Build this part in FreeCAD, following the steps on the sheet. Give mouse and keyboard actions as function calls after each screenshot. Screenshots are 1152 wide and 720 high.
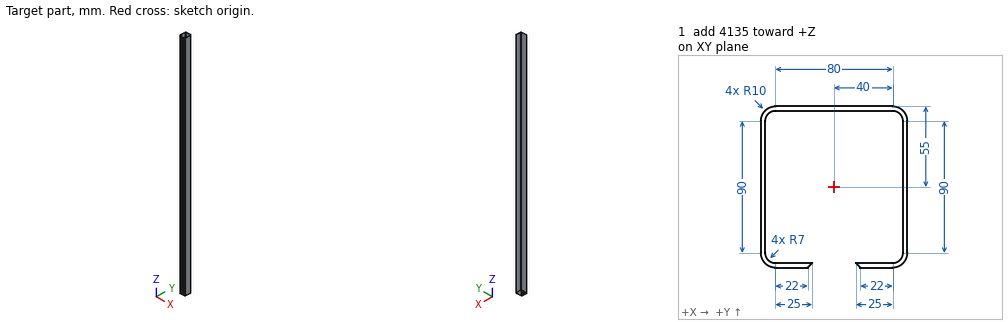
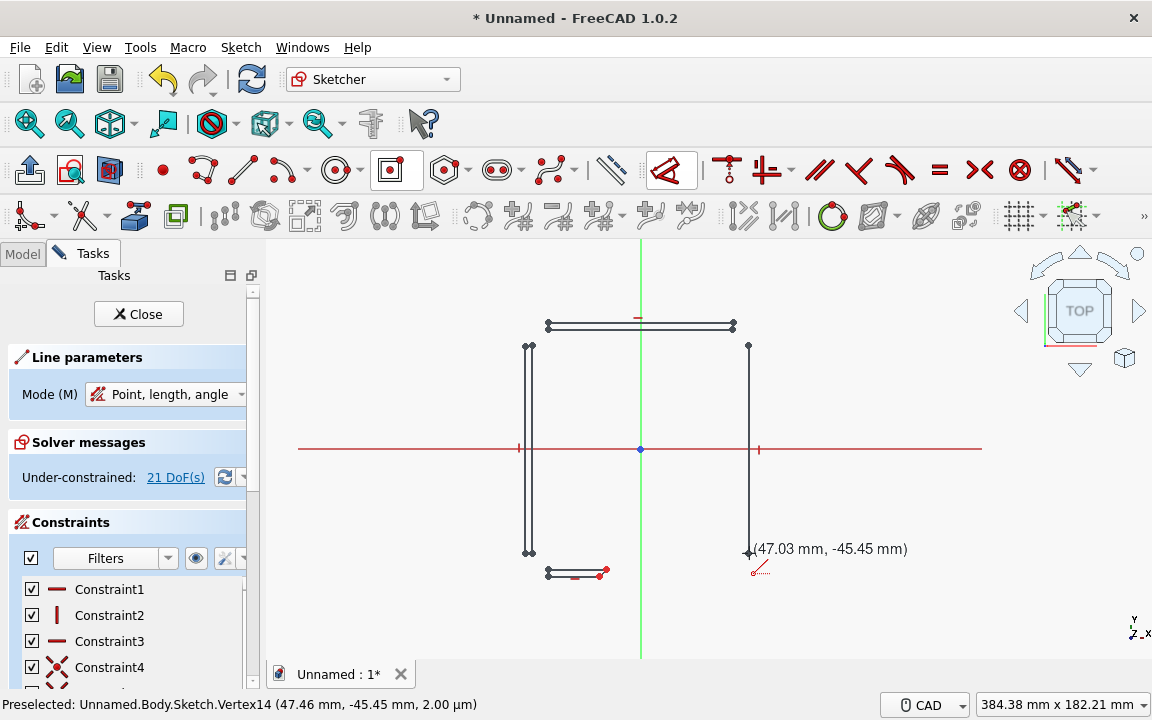
click(204, 170)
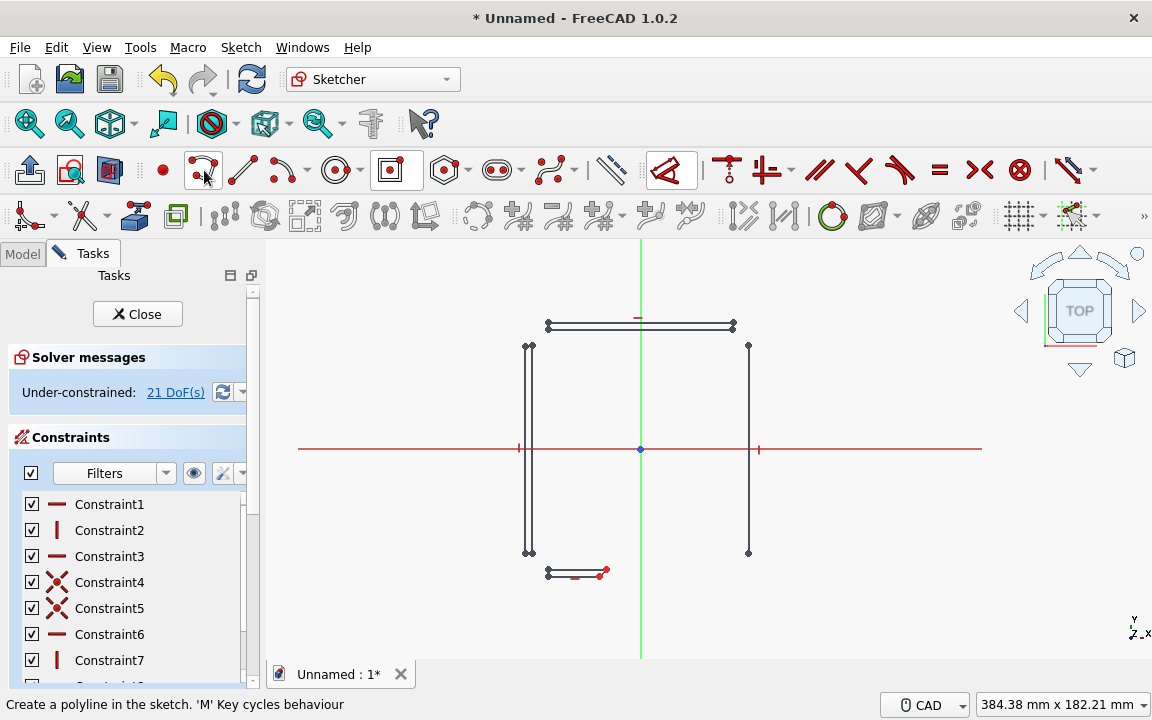
click(733, 569)
click(675, 569)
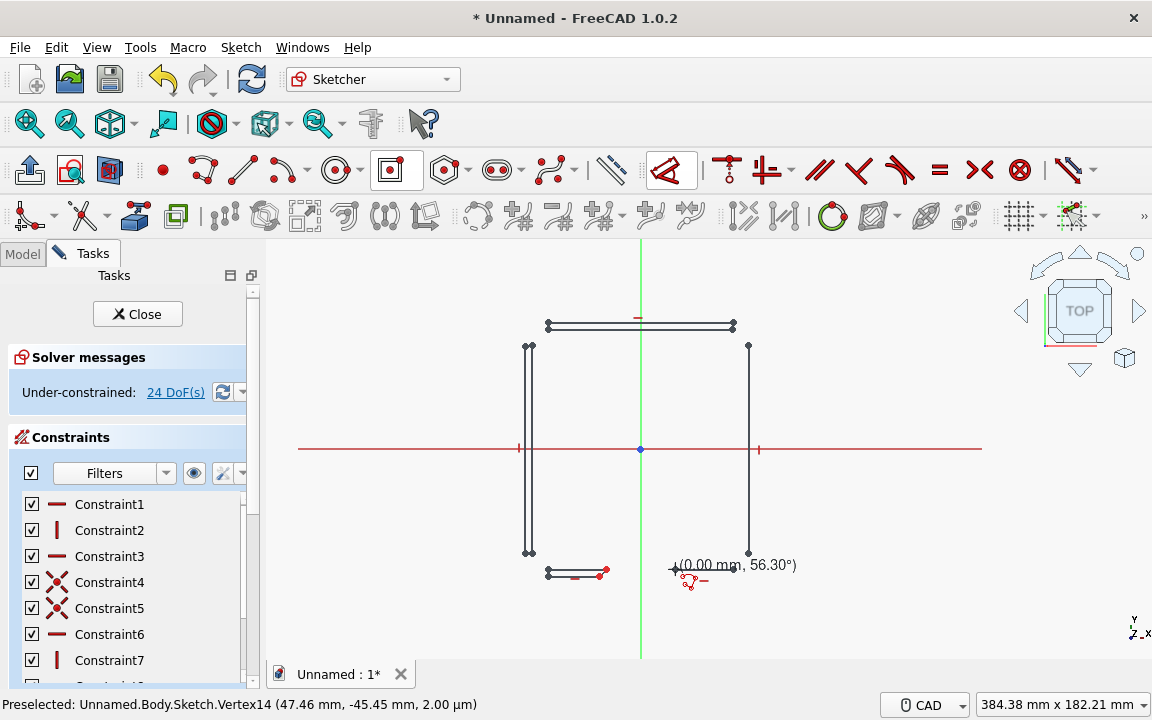
scroll(682, 576, up, 5)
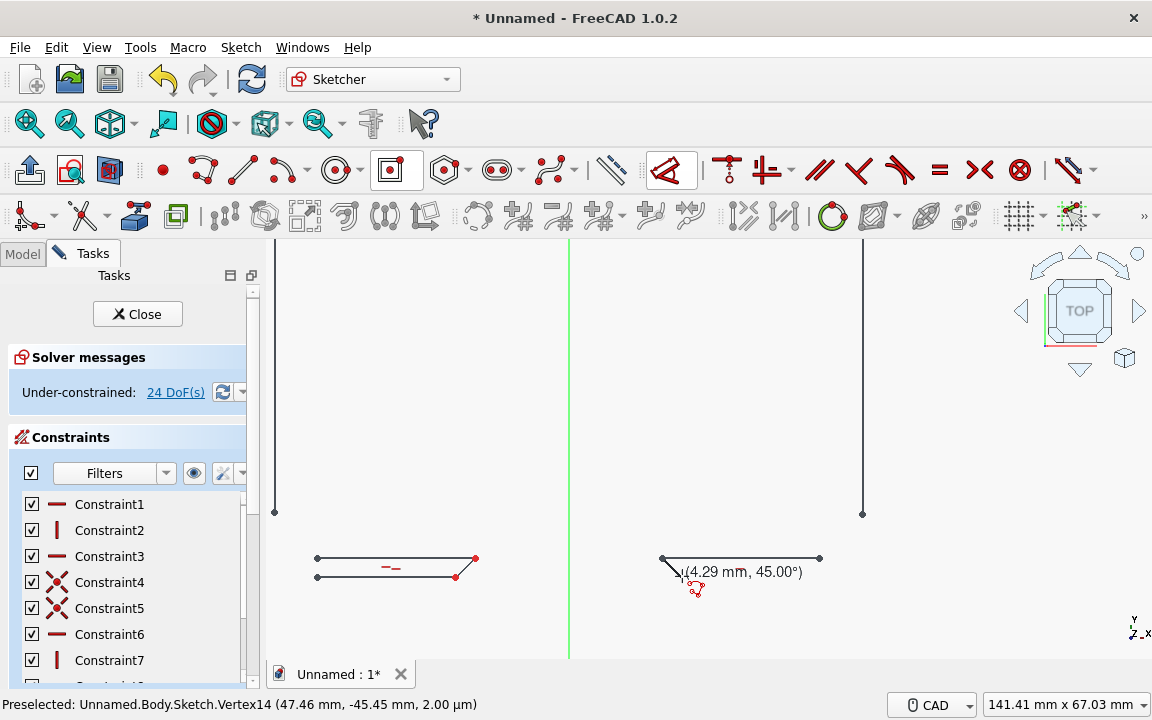
click(681, 575)
click(819, 575)
right_click(819, 575)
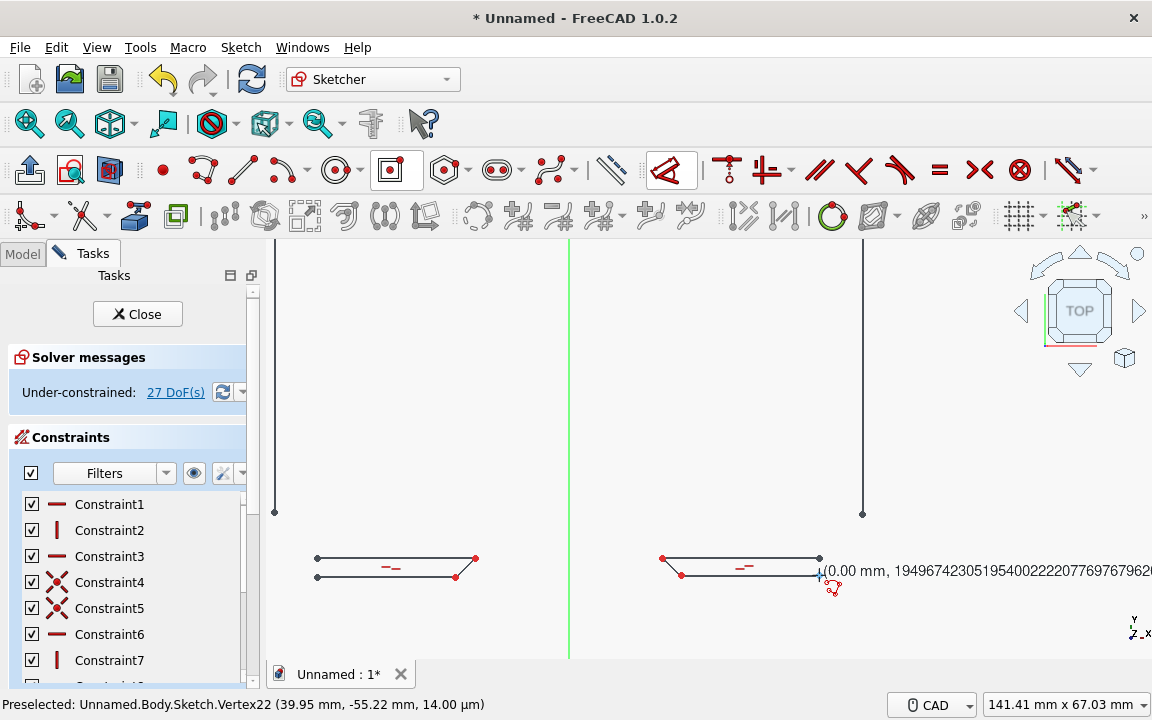
click(244, 170)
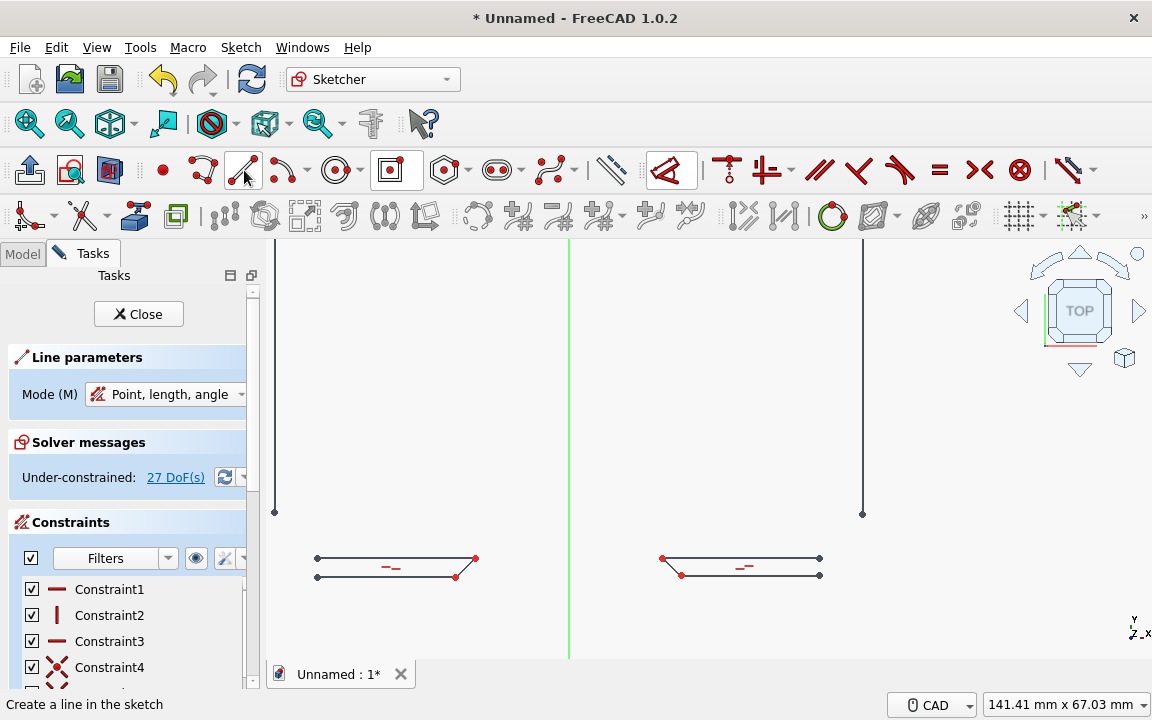
click(882, 512)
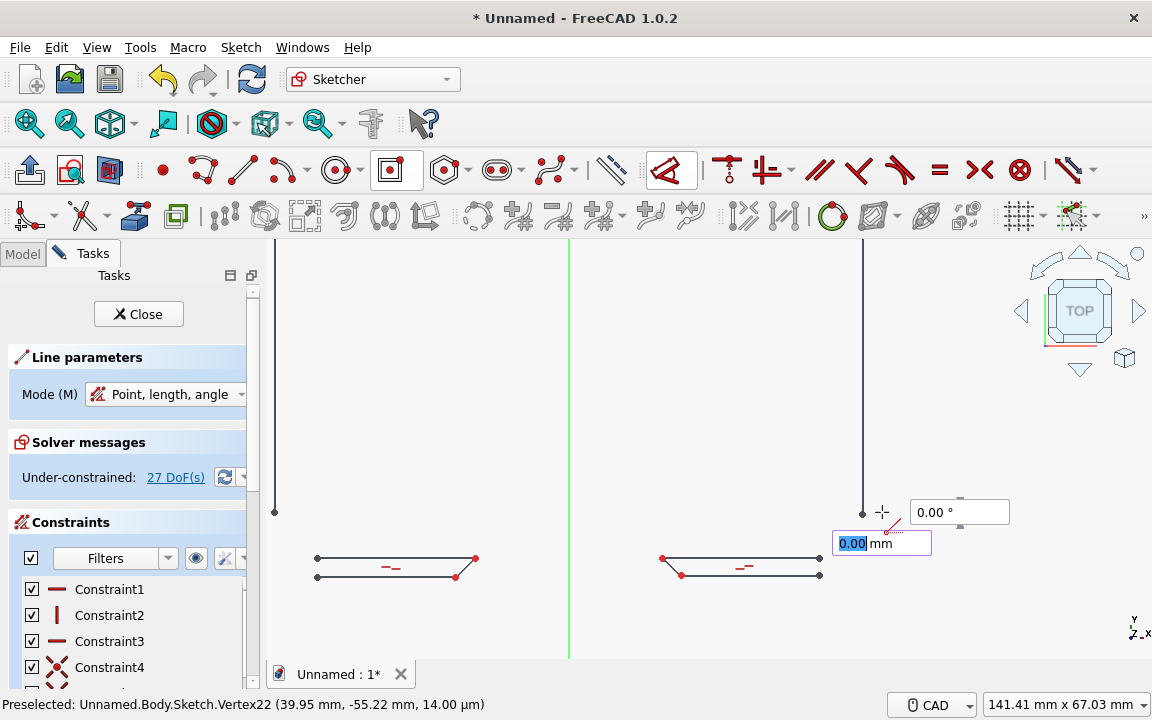
scroll(682, 576, down, 5)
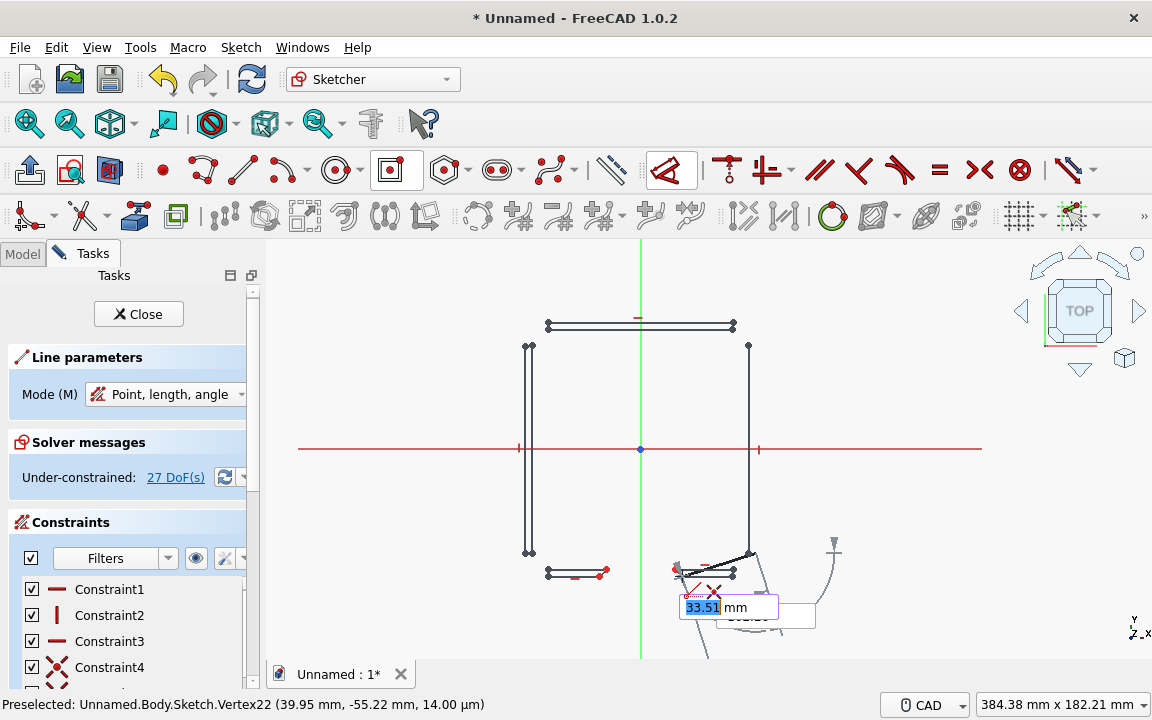
scroll(756, 346, up, 5)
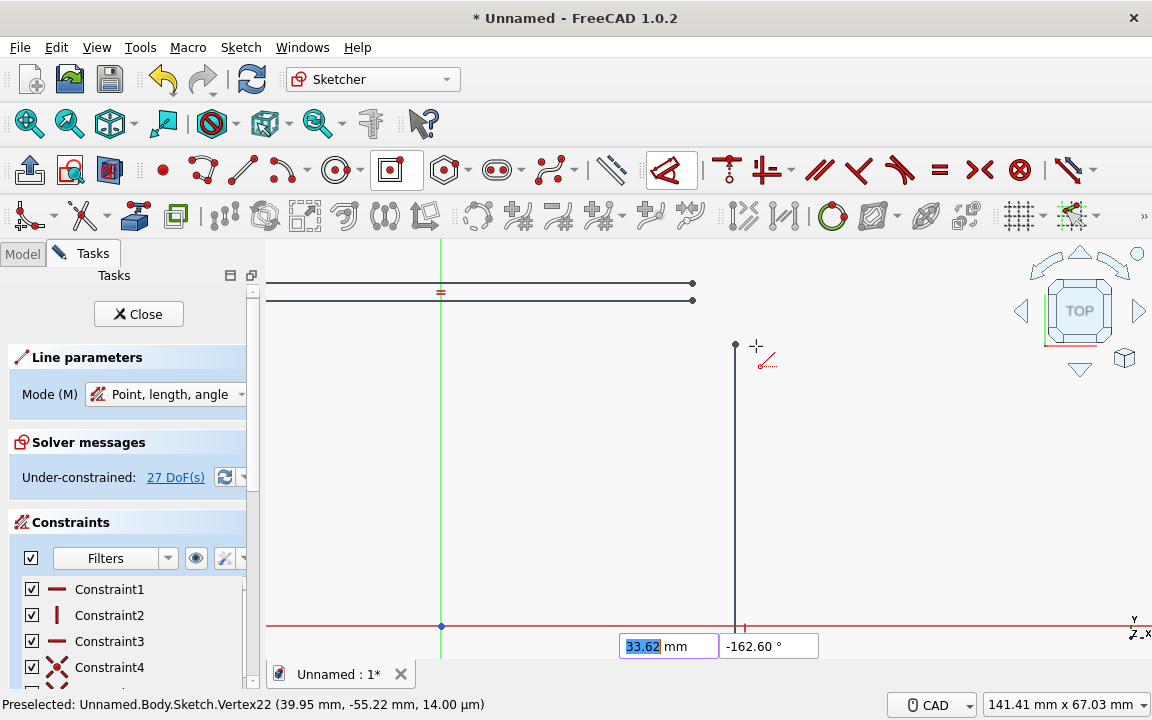
click(755, 344)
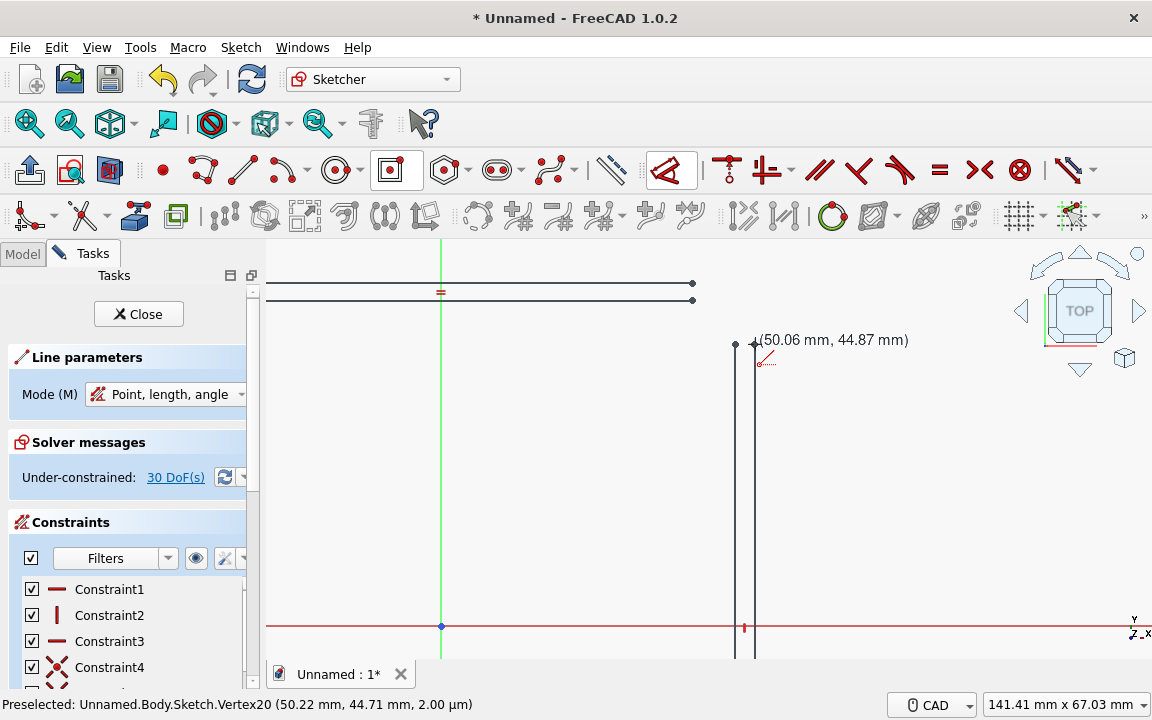
click(310, 170)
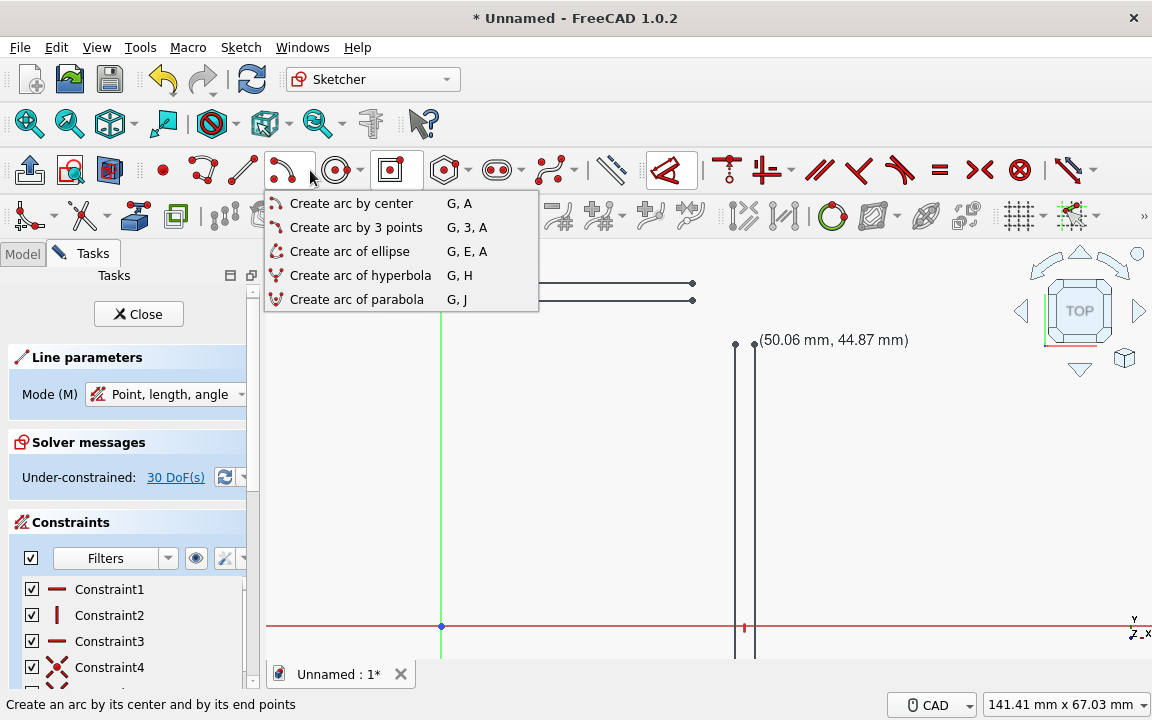
click(402, 227)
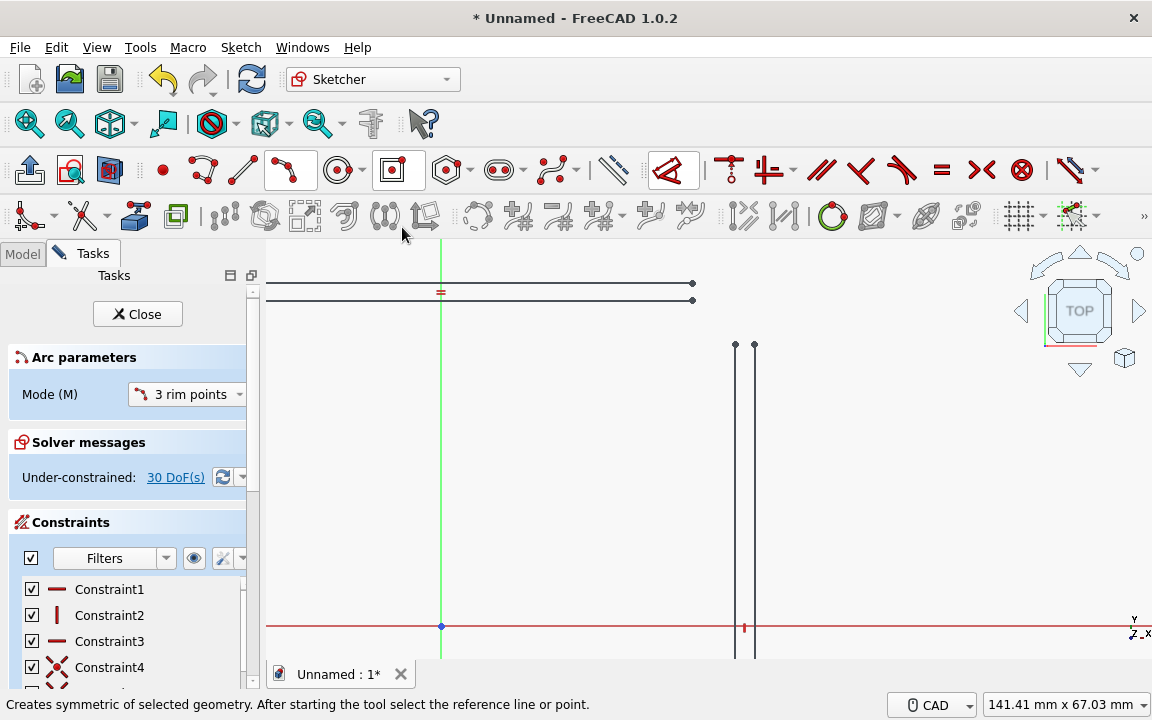
scroll(756, 346, down, 5)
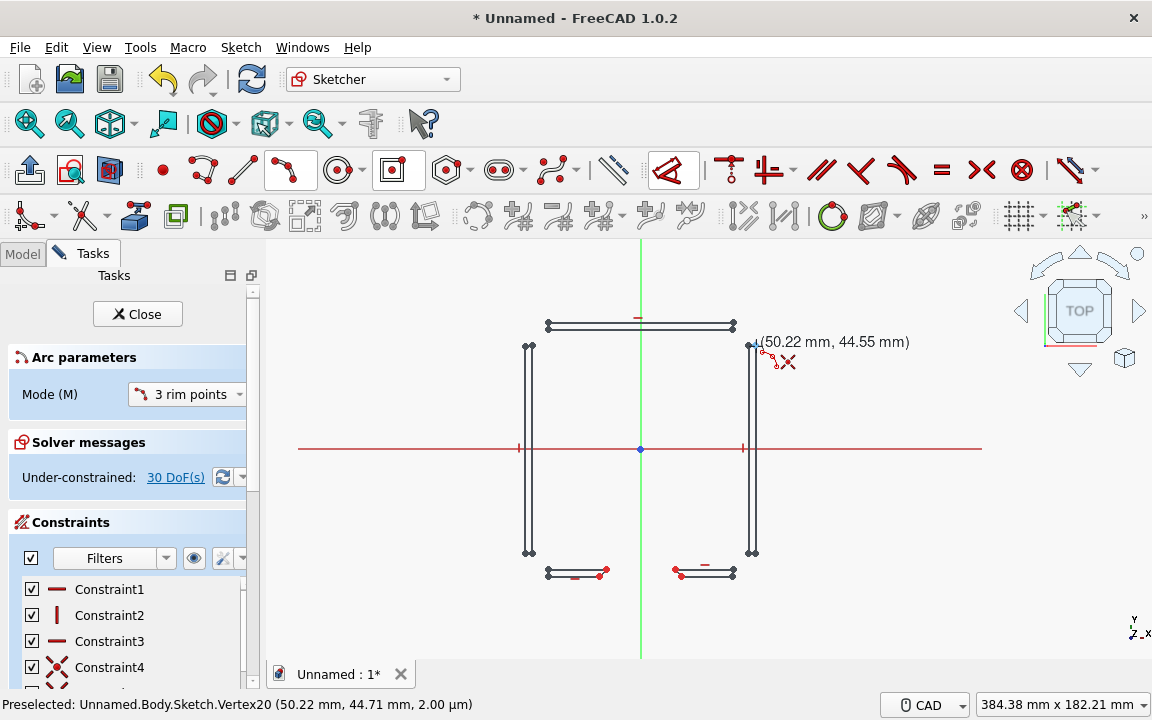
scroll(548, 322, up, 5)